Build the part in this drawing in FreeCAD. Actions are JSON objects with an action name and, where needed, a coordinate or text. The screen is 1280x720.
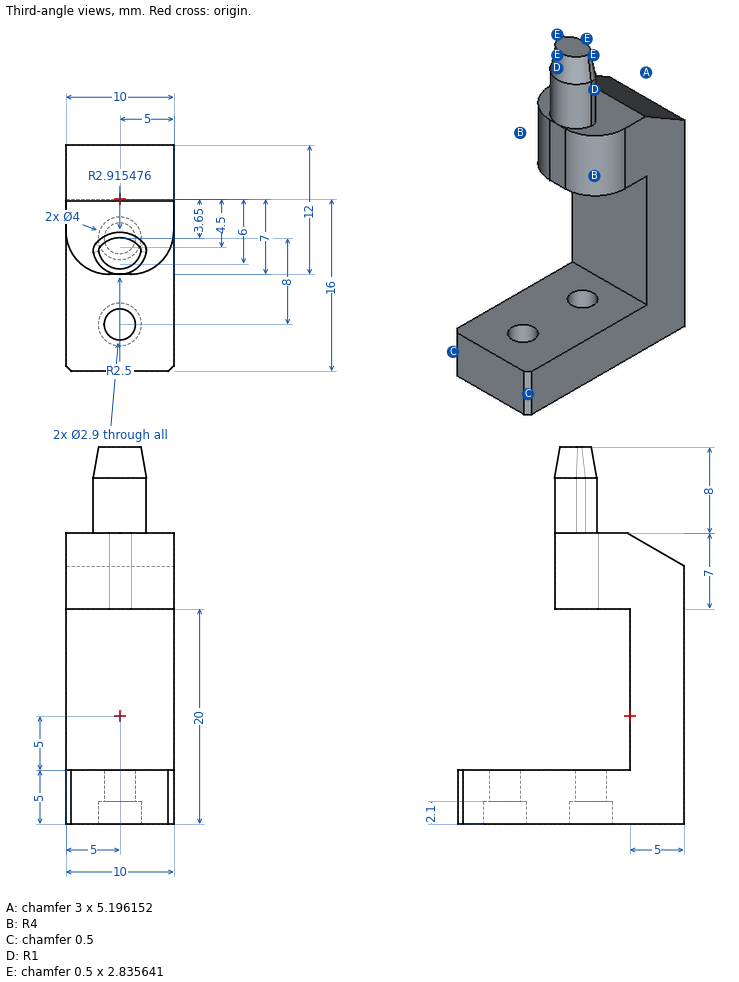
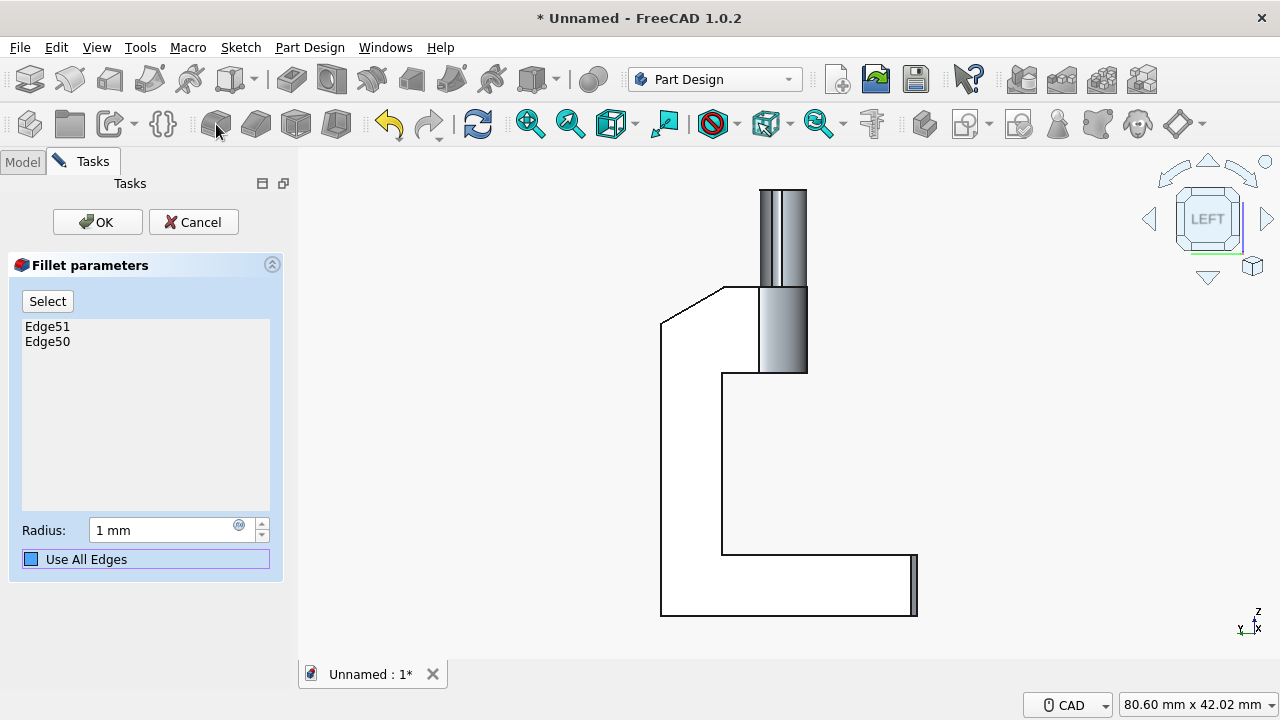
{"action": "left_click", "coordinate": [98, 222]}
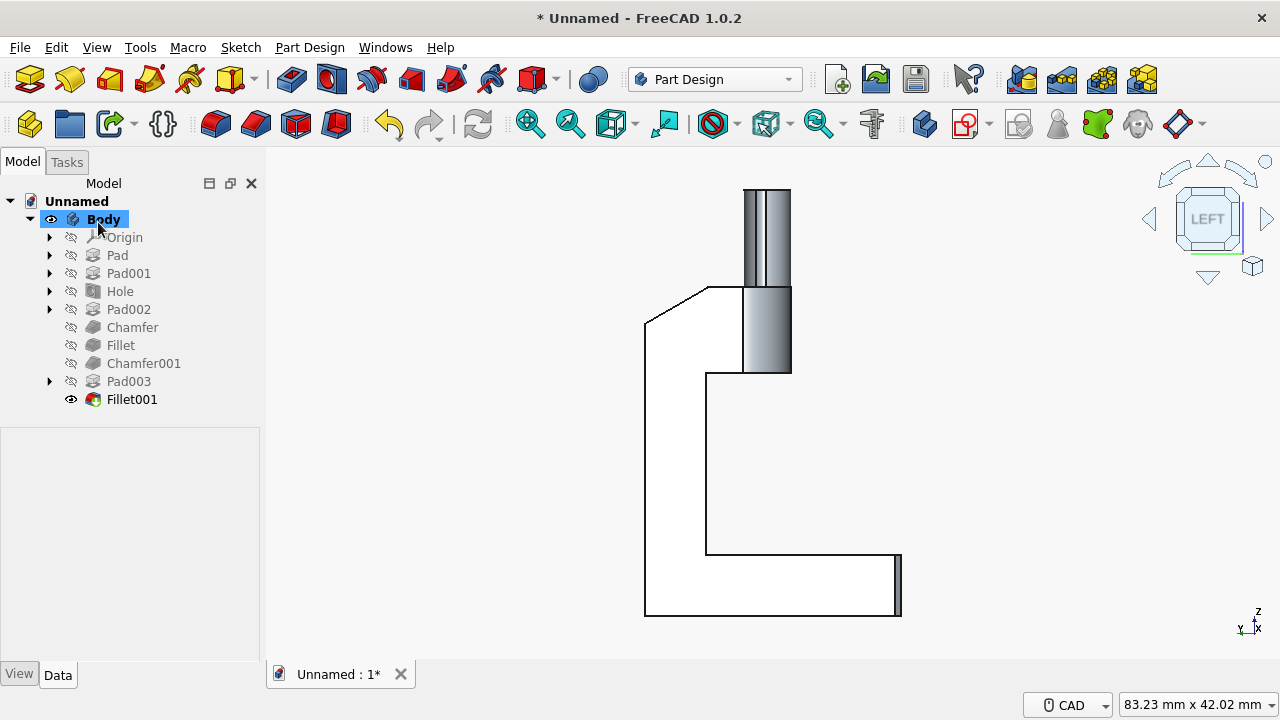
{"action": "key", "text": "0"}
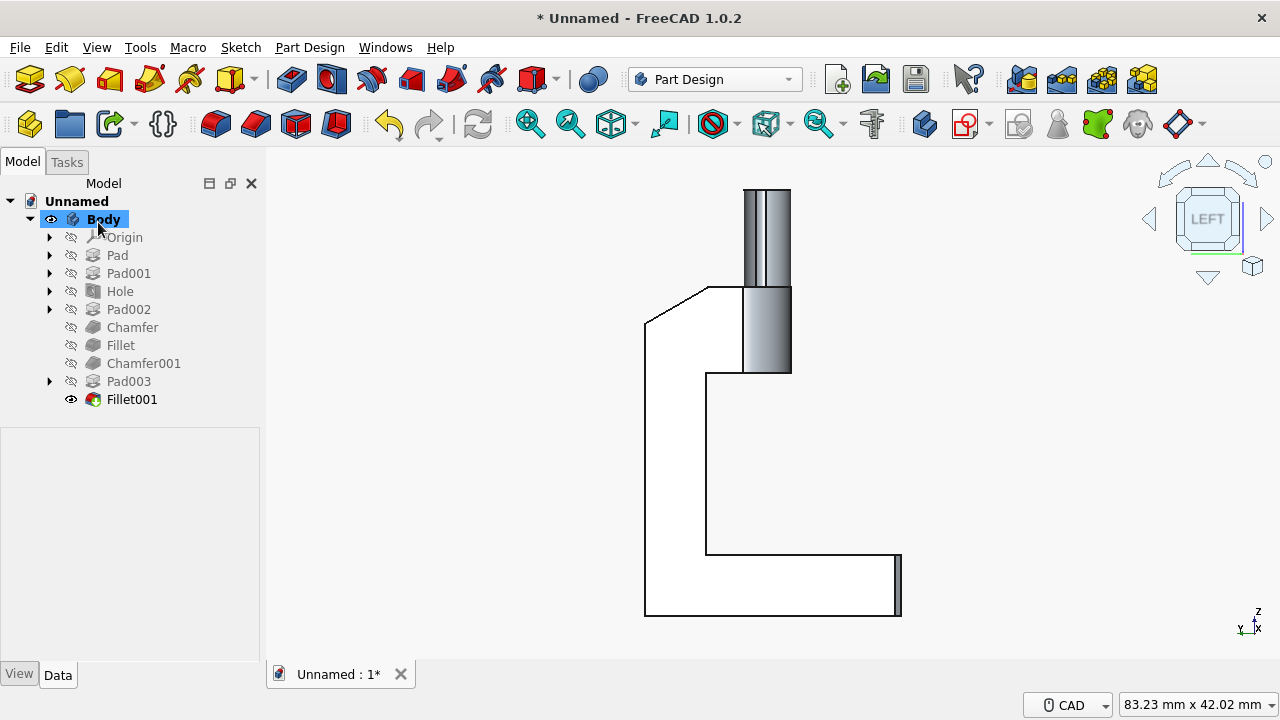
{"action": "left_click", "coordinate": [777, 226]}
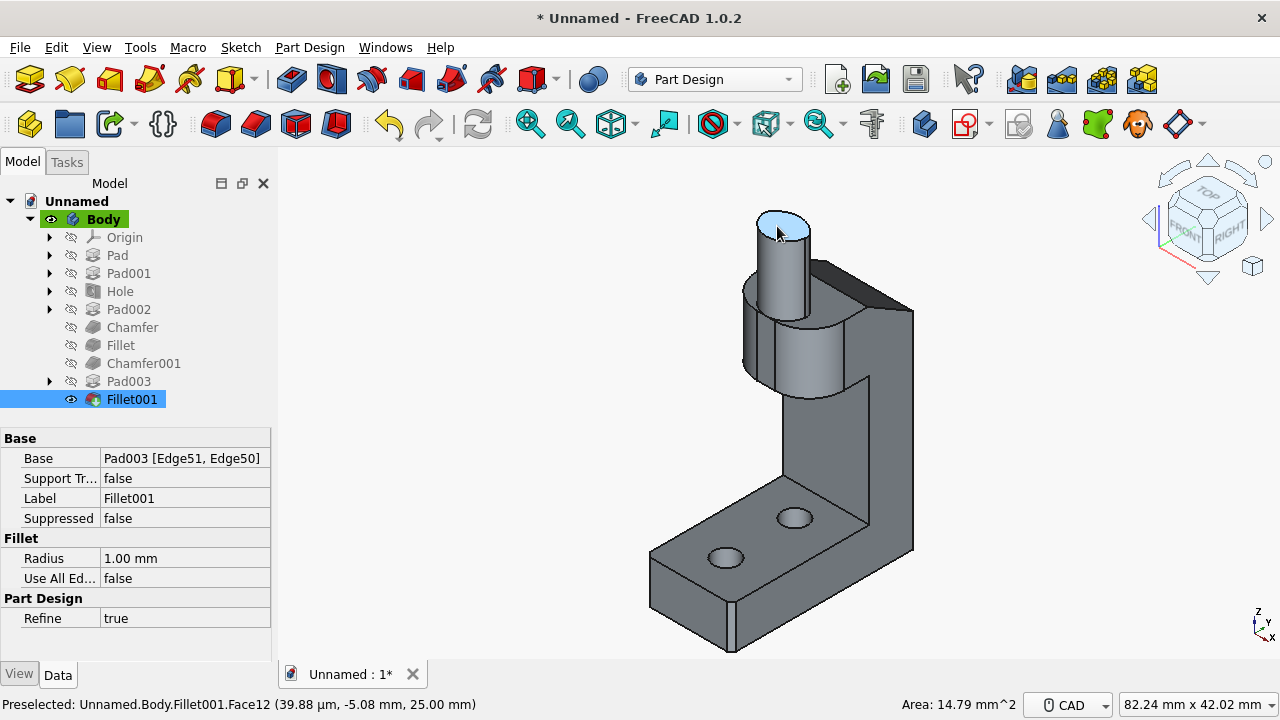
{"action": "left_click", "coordinate": [256, 124]}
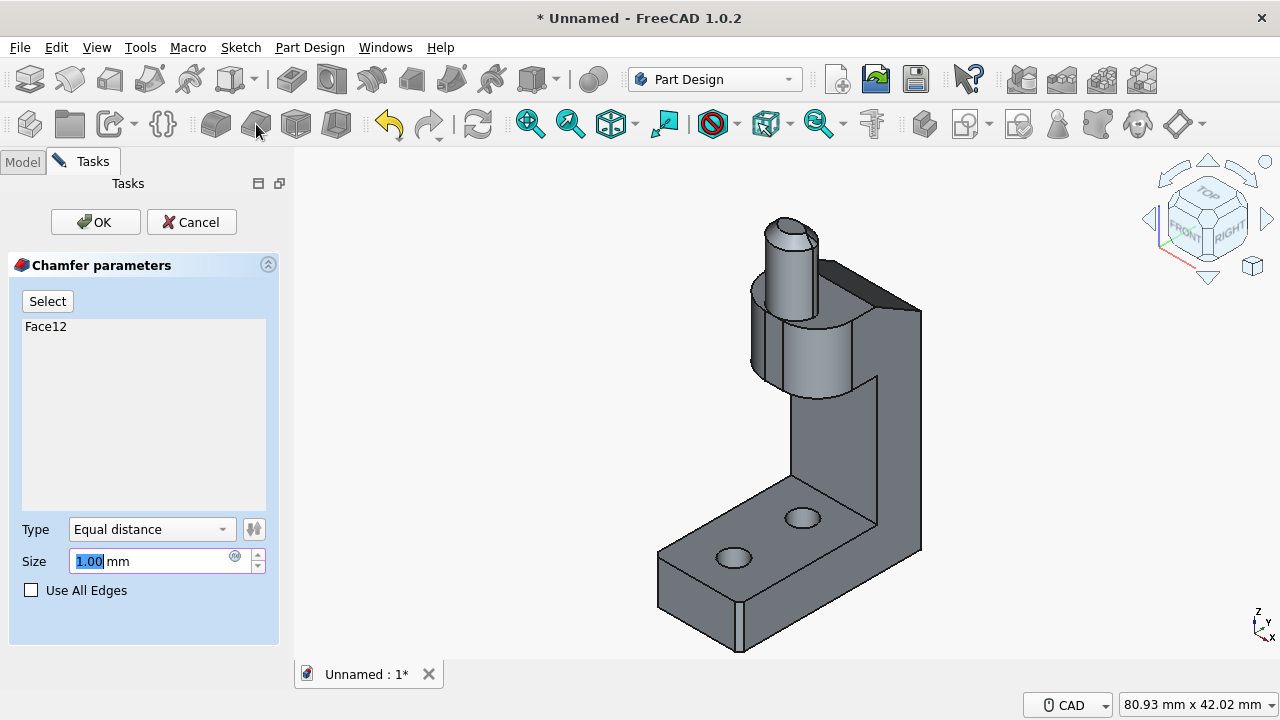
{"action": "type", "text": "0.5"}
{"action": "key", "text": "Tab"}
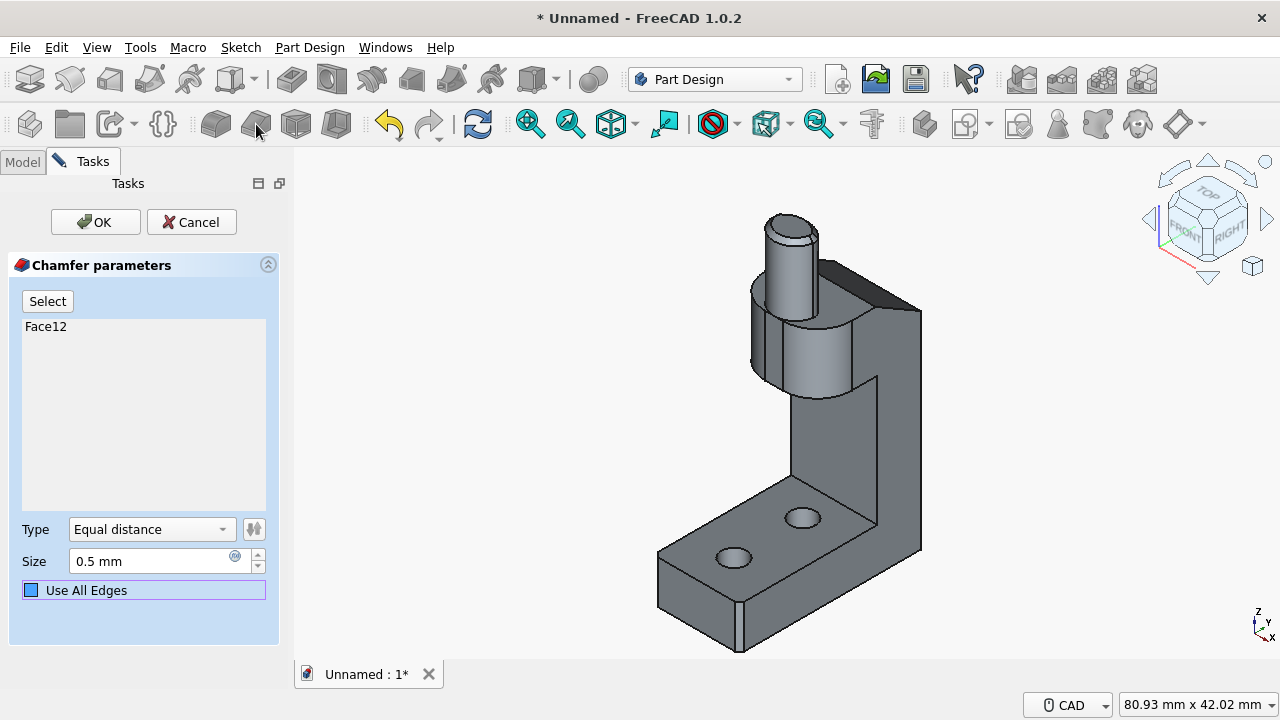
{"action": "left_click", "coordinate": [153, 530]}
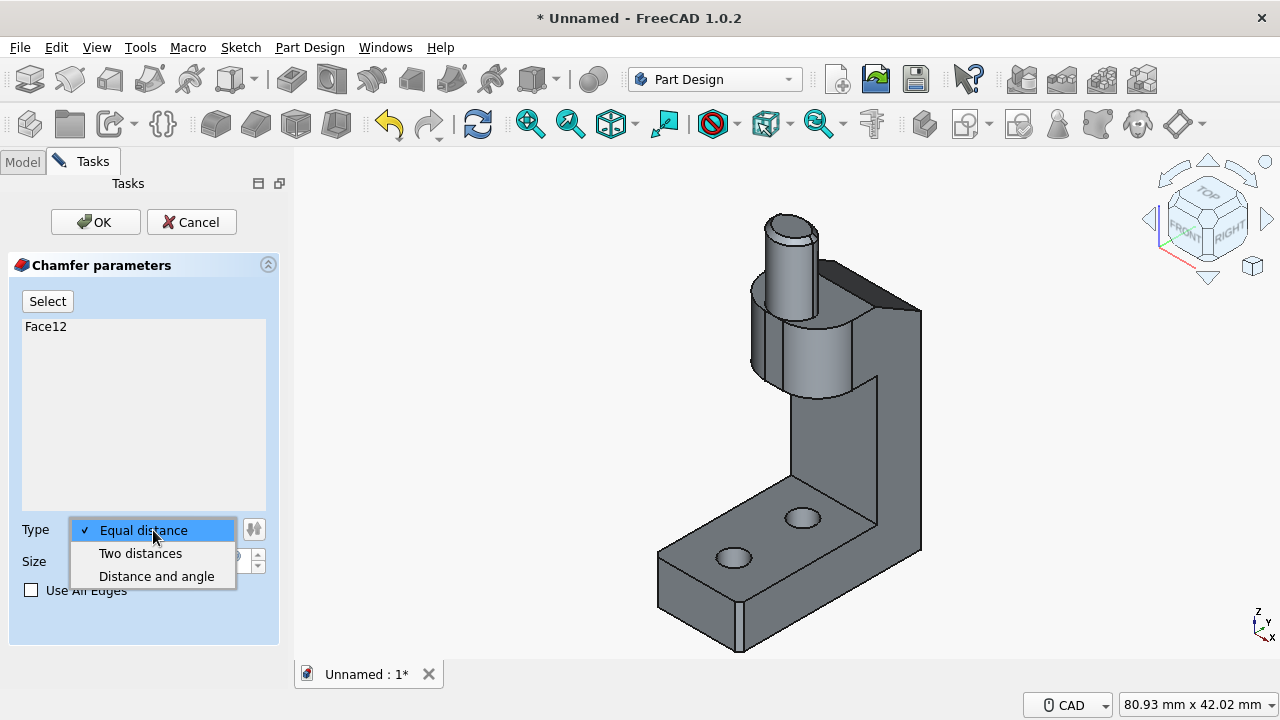
{"action": "left_click", "coordinate": [152, 554]}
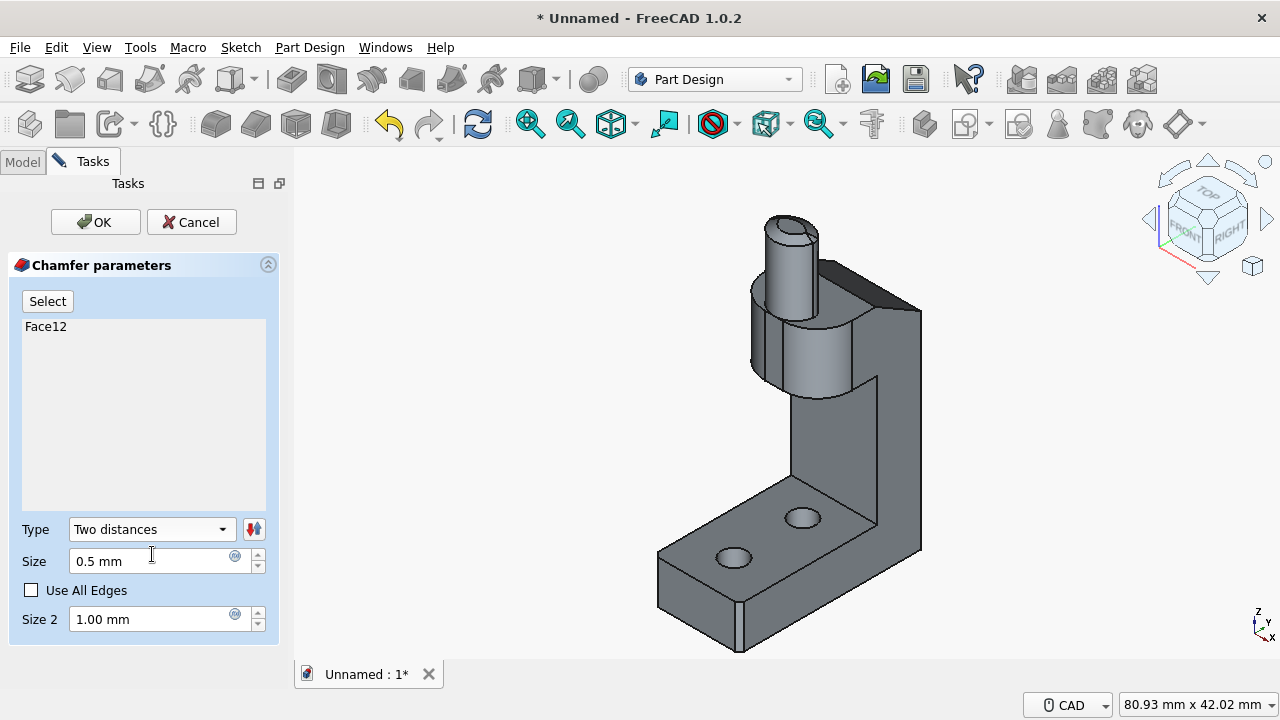
{"action": "triple_click", "coordinate": [160, 619]}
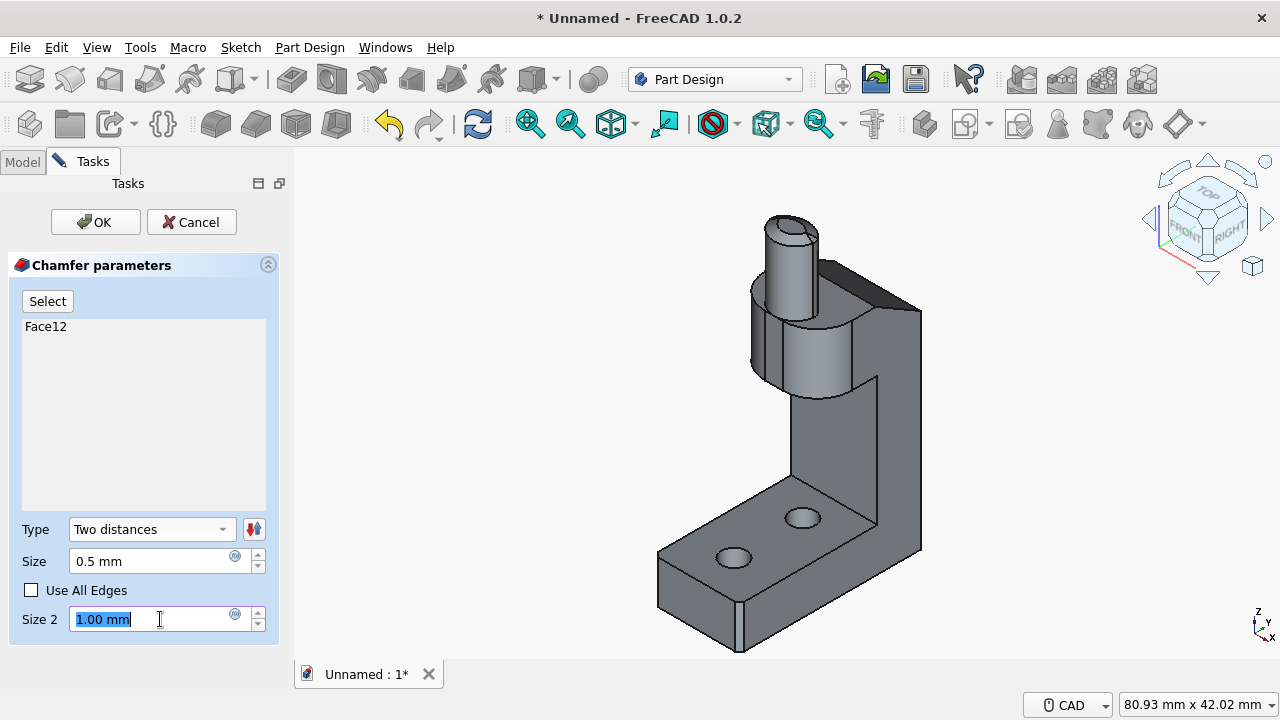
{"action": "type", "text": "2.835641"}
{"action": "key", "text": "Tab"}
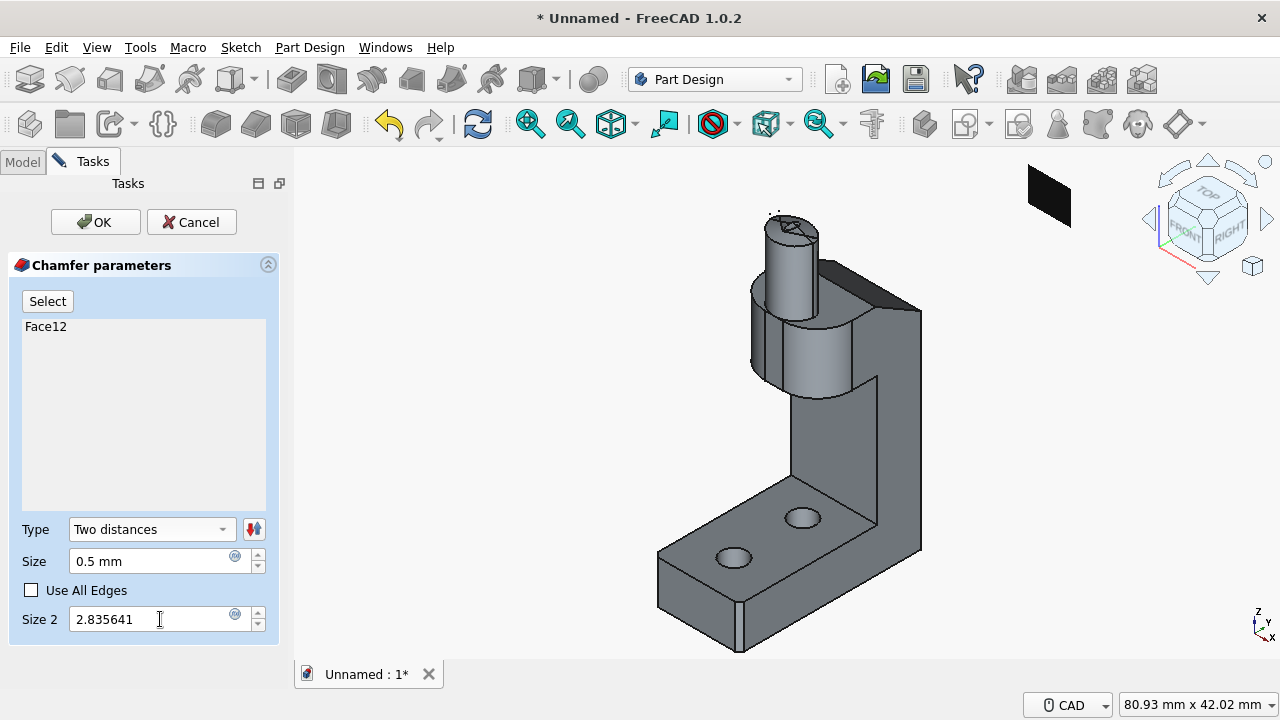
{"action": "left_click", "coordinate": [254, 530]}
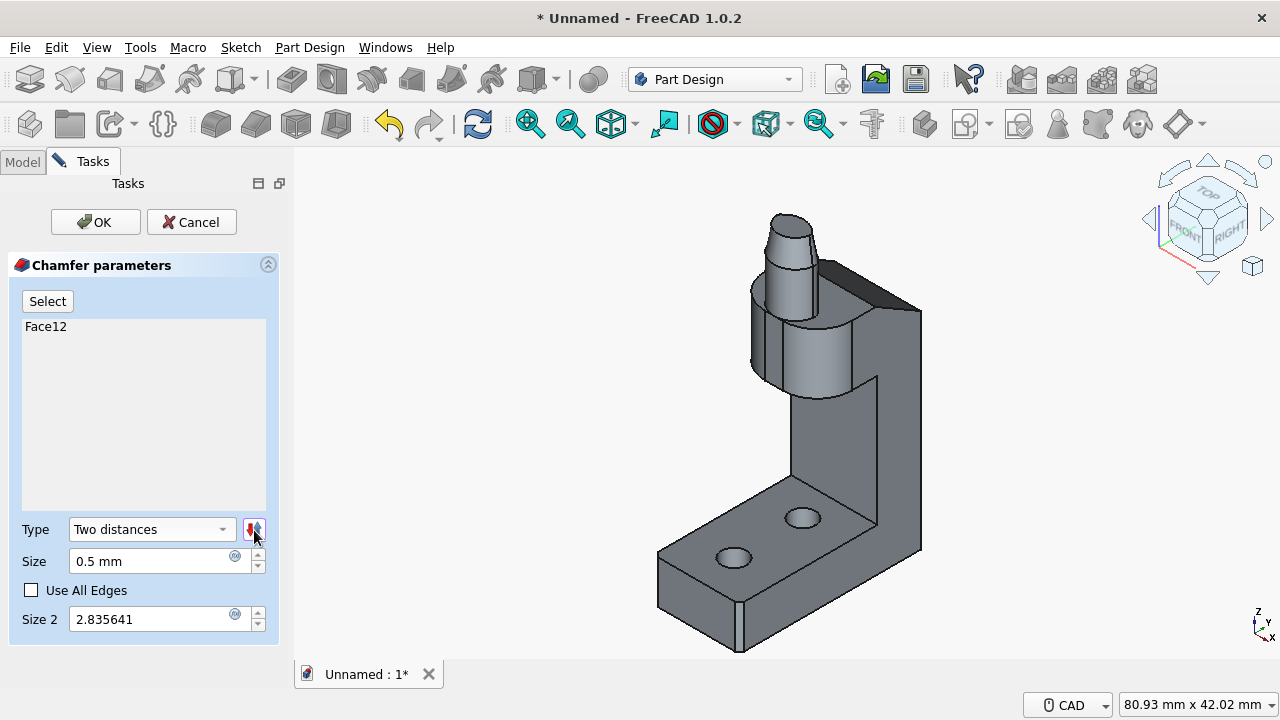
{"action": "left_click", "coordinate": [96, 222]}